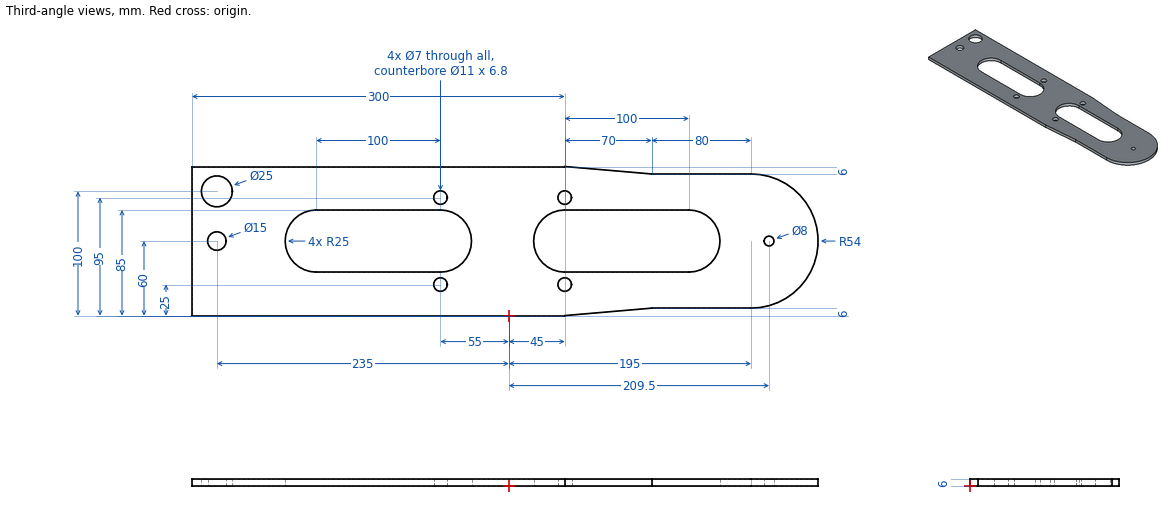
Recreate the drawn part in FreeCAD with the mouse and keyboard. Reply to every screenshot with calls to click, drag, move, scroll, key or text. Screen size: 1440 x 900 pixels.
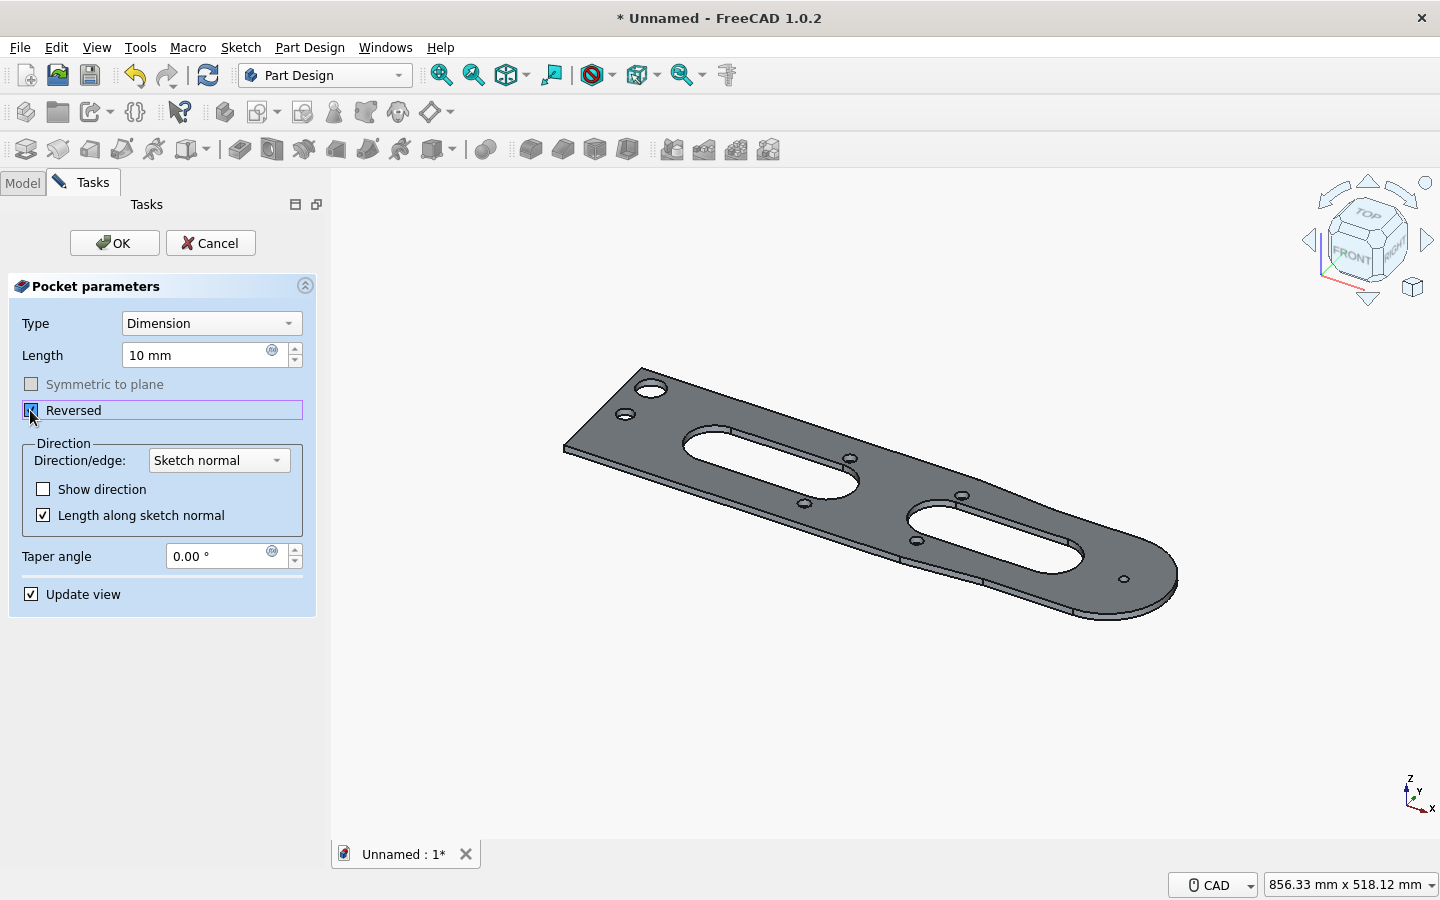
click(115, 243)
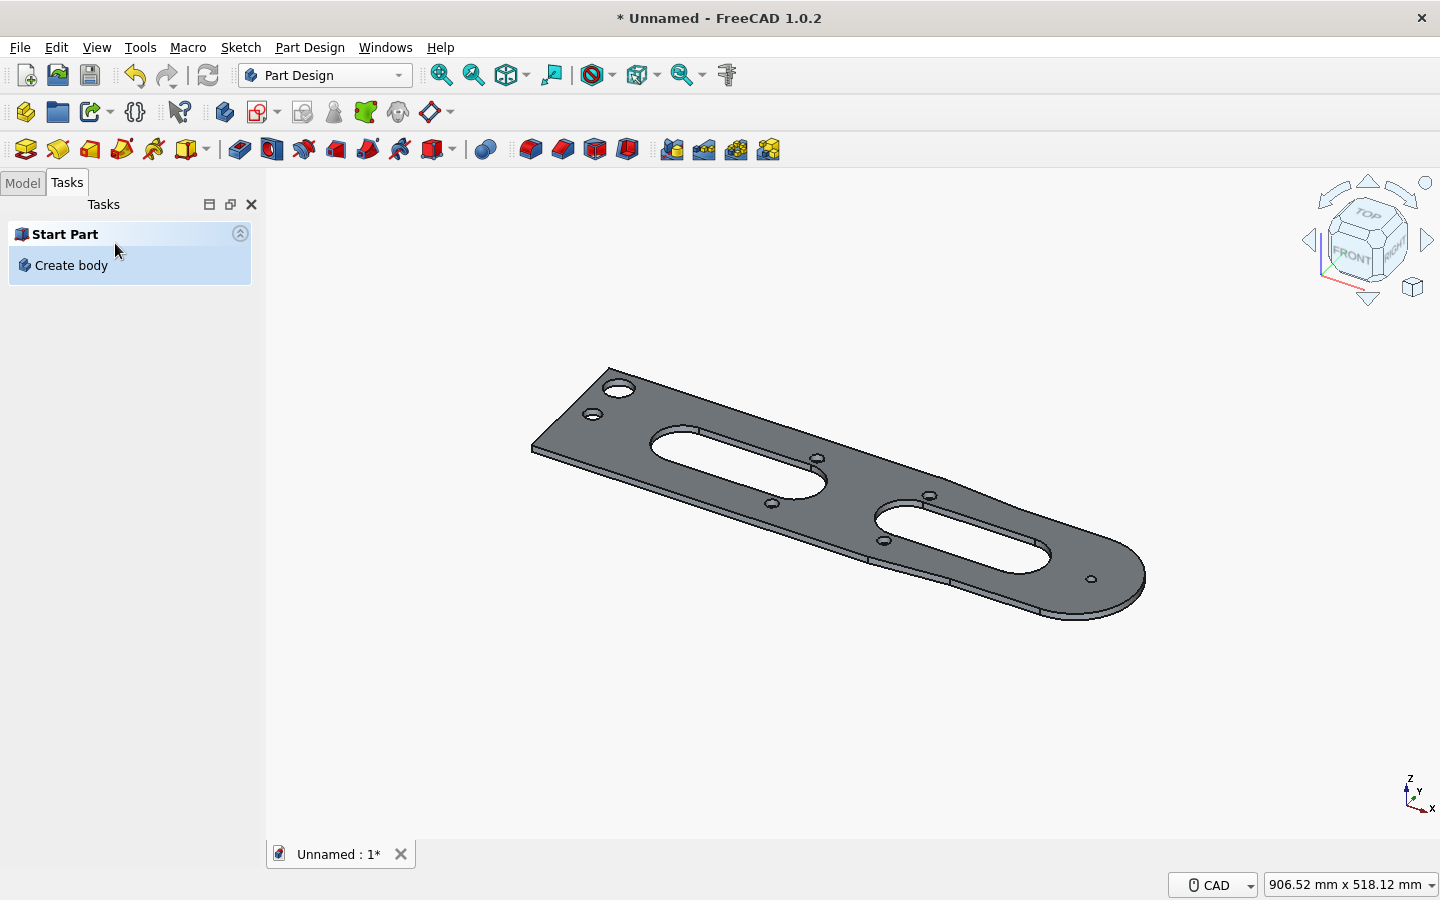
key(0)